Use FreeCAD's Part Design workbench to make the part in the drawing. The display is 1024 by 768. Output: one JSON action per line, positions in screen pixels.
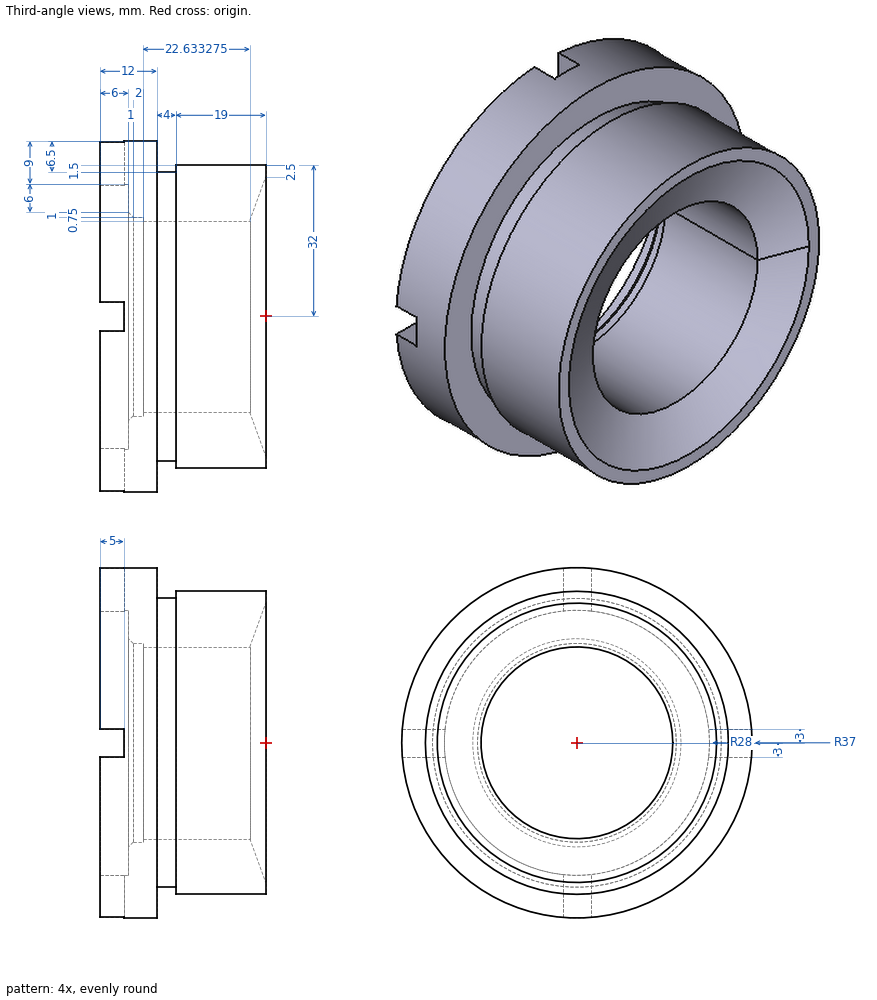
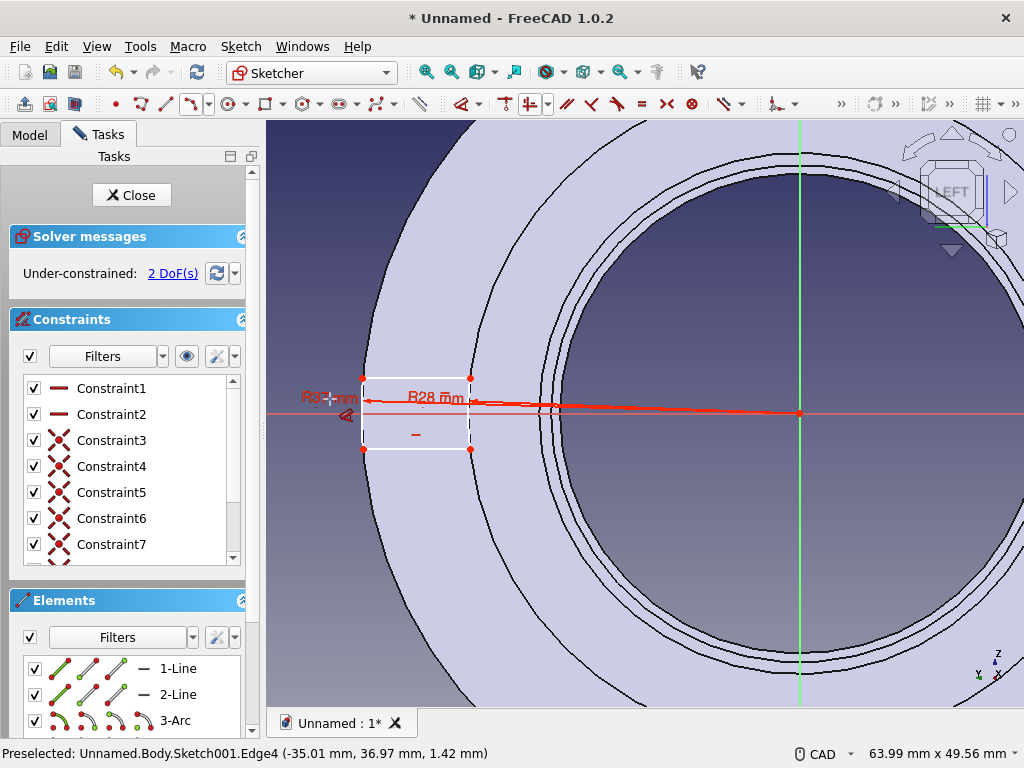
{"action": "left_click", "coordinate": [363, 449]}
{"action": "left_click", "coordinate": [834, 432]}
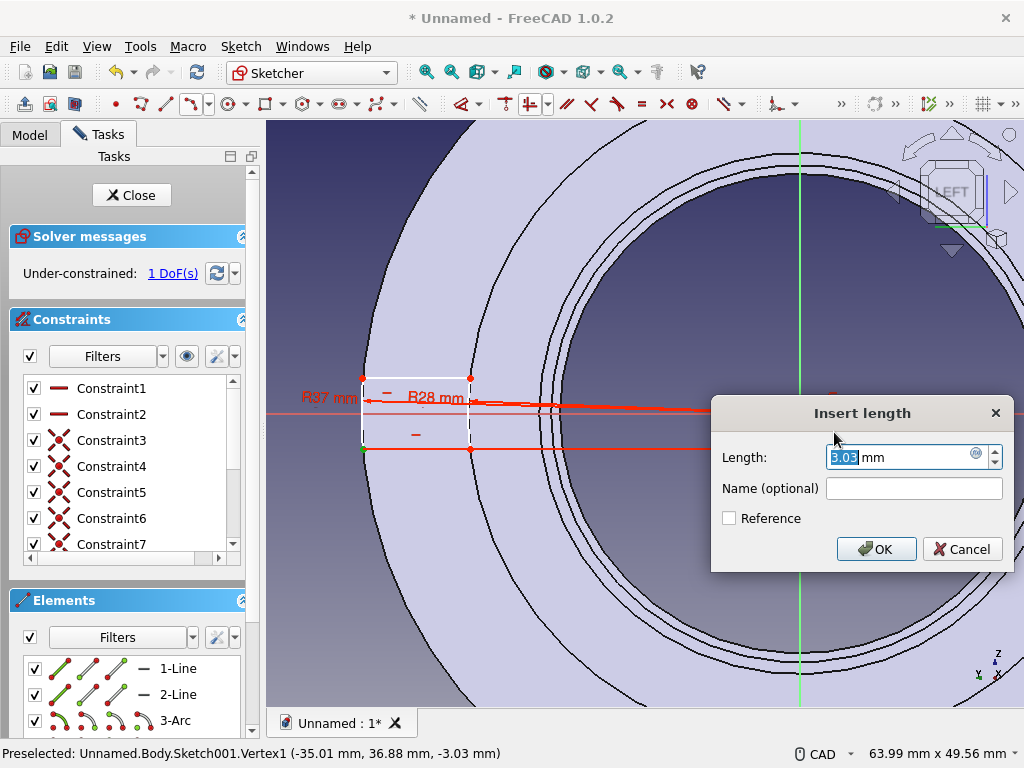
{"action": "type", "text": "3"}
{"action": "key", "text": "Return"}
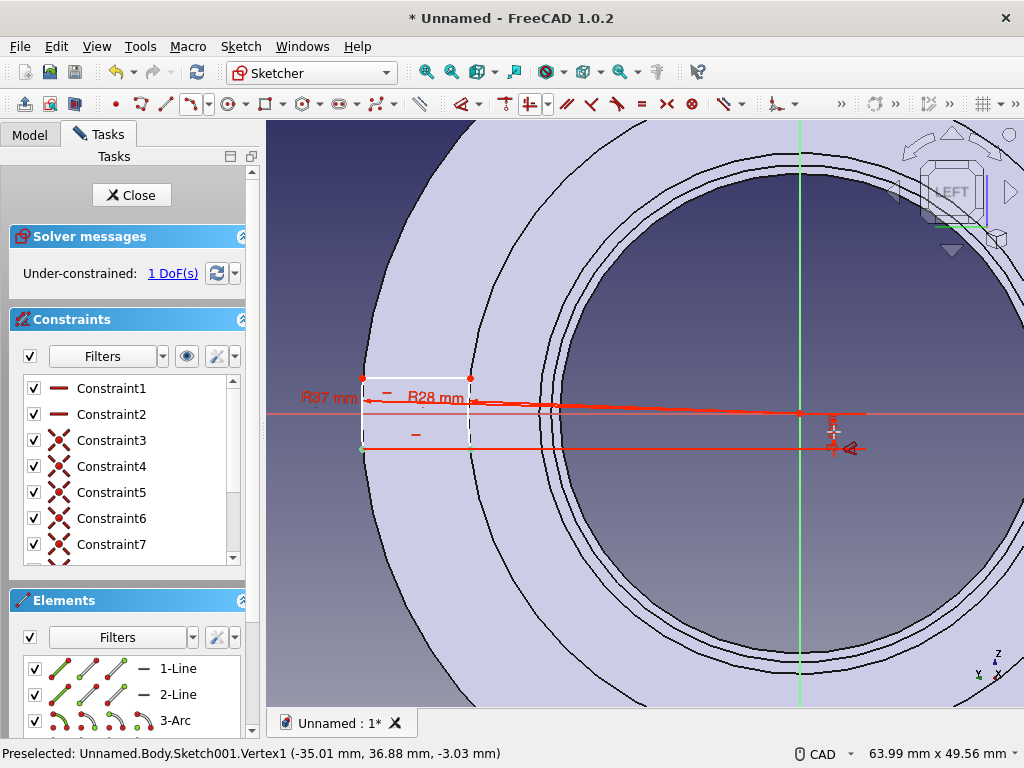
{"action": "left_click", "coordinate": [470, 378]}
{"action": "left_click", "coordinate": [834, 396]}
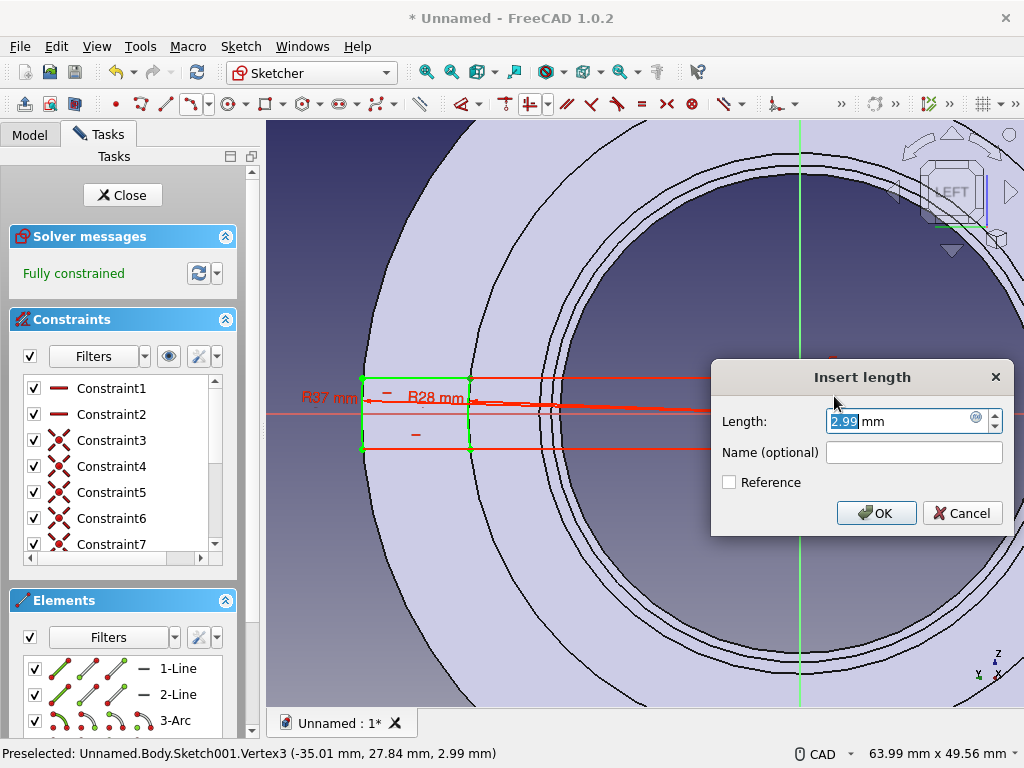
{"action": "type", "text": "3"}
{"action": "key", "text": "Return"}
{"action": "key", "text": "Escape"}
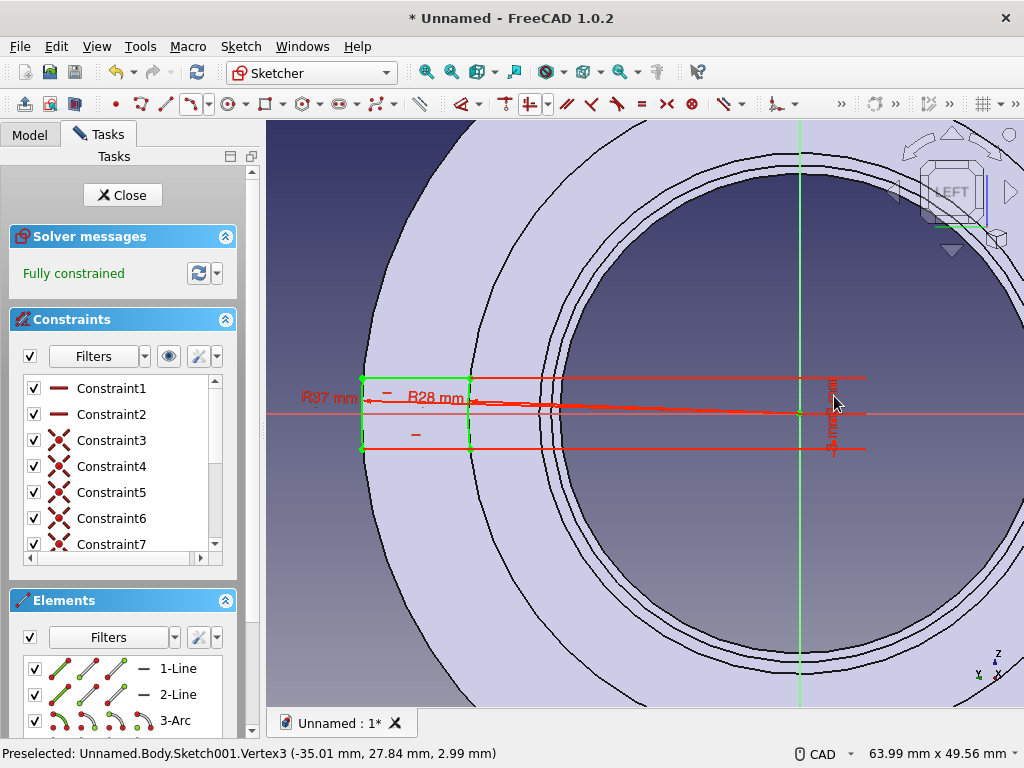
{"action": "left_click", "coordinate": [123, 195]}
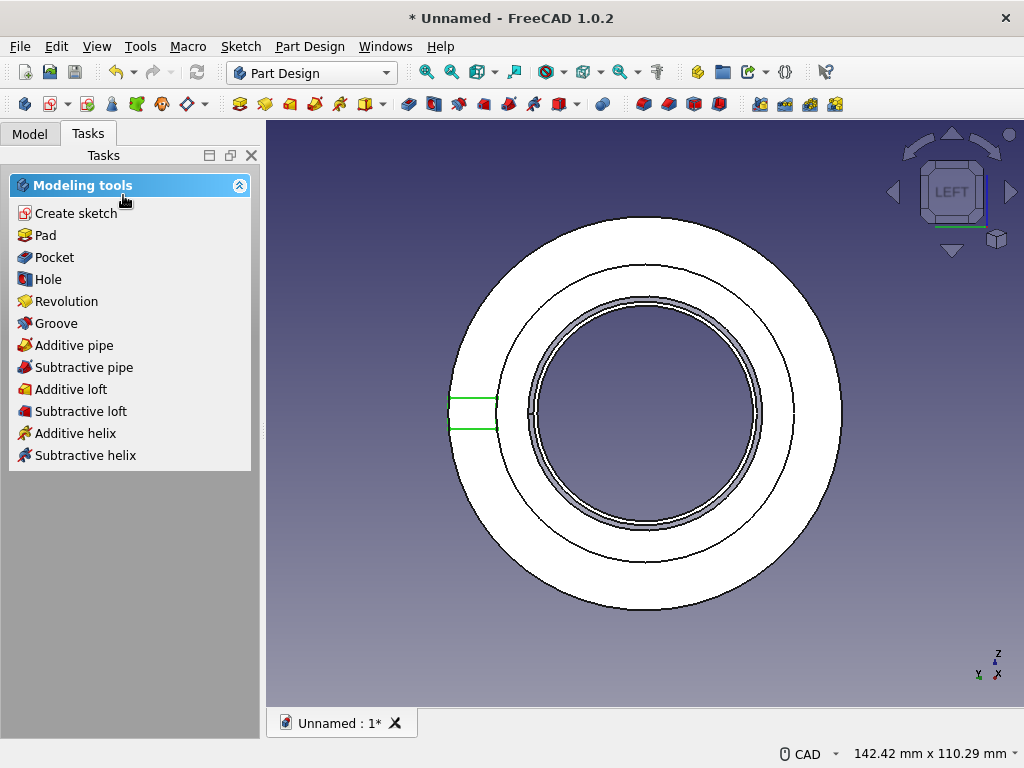
{"action": "left_click", "coordinate": [409, 104]}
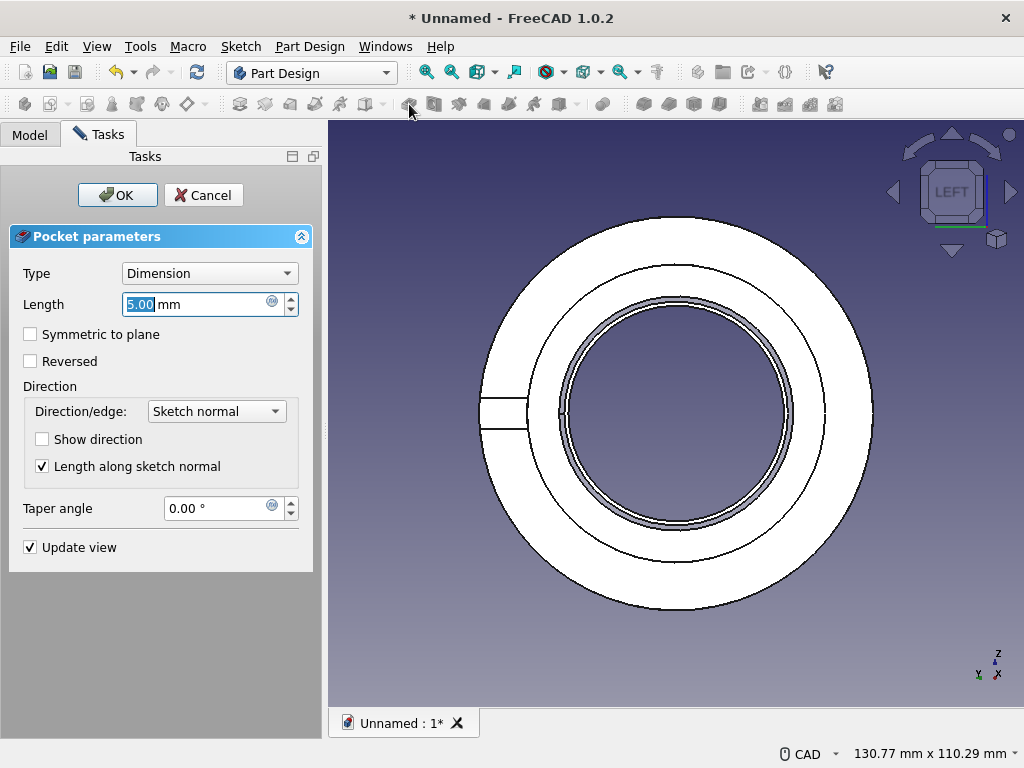
{"action": "type", "text": "5"}
{"action": "key", "text": "Tab"}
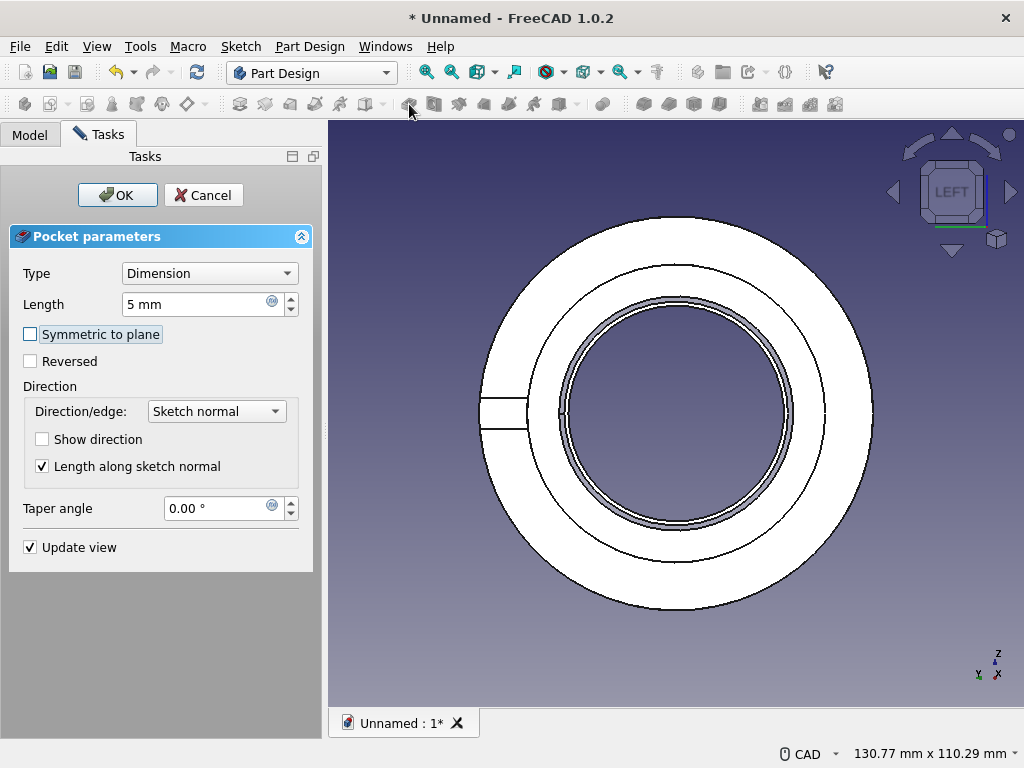
{"action": "left_click", "coordinate": [118, 195]}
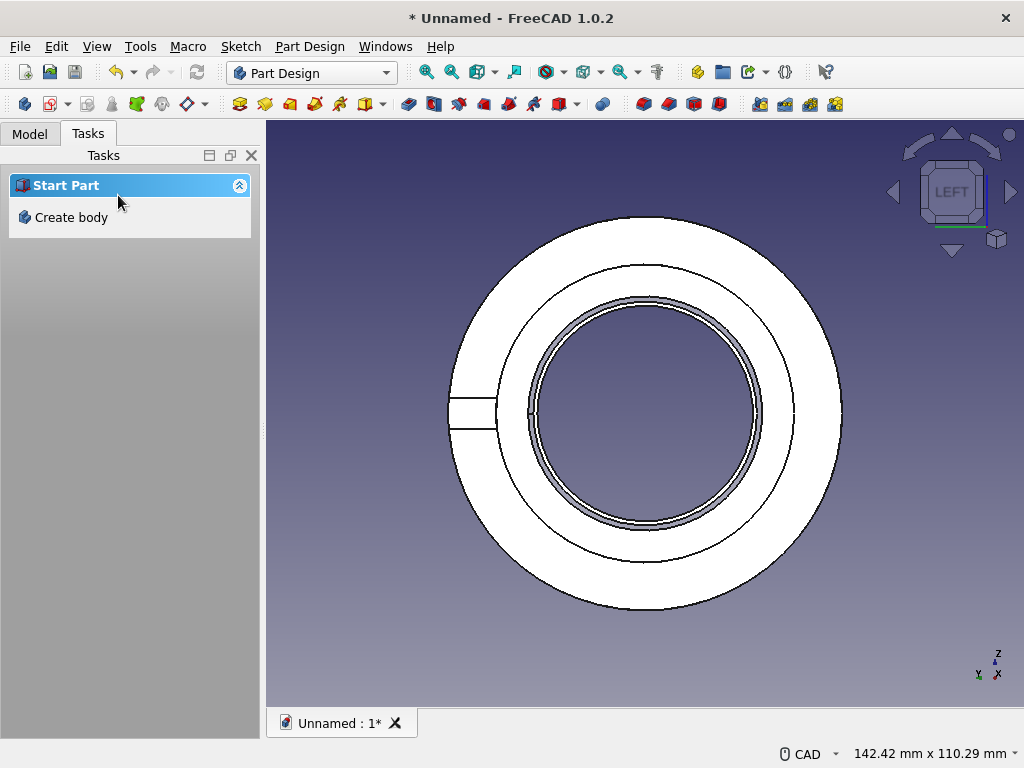
{"action": "left_click", "coordinate": [30, 134]}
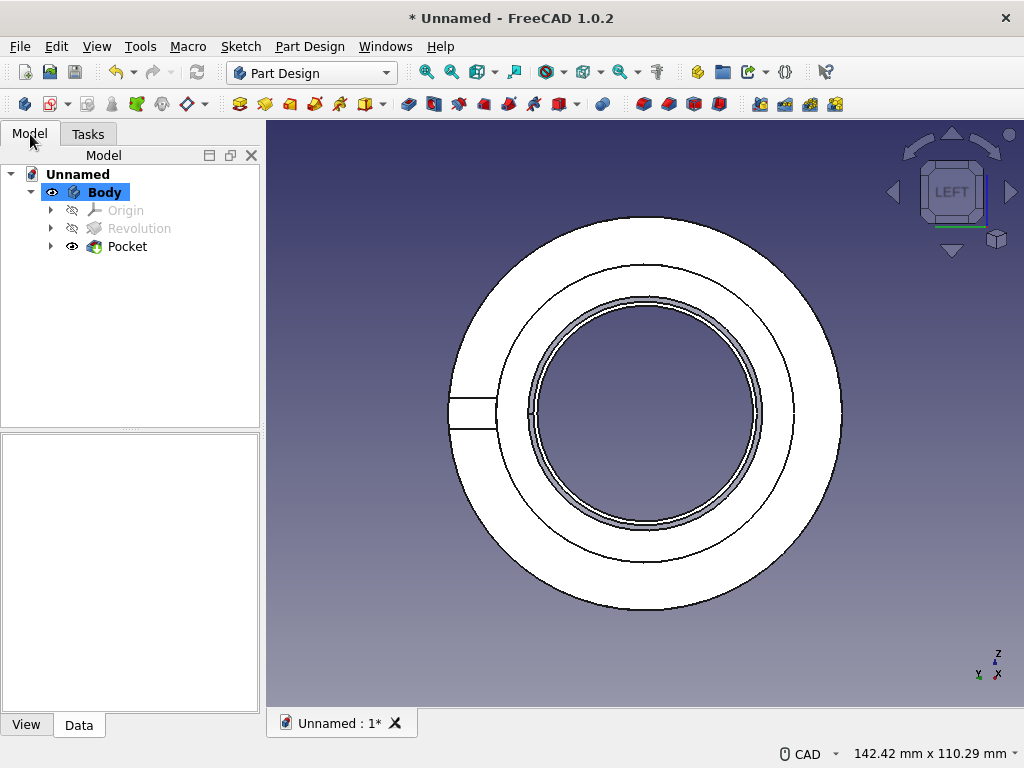
{"action": "left_click", "coordinate": [117, 246]}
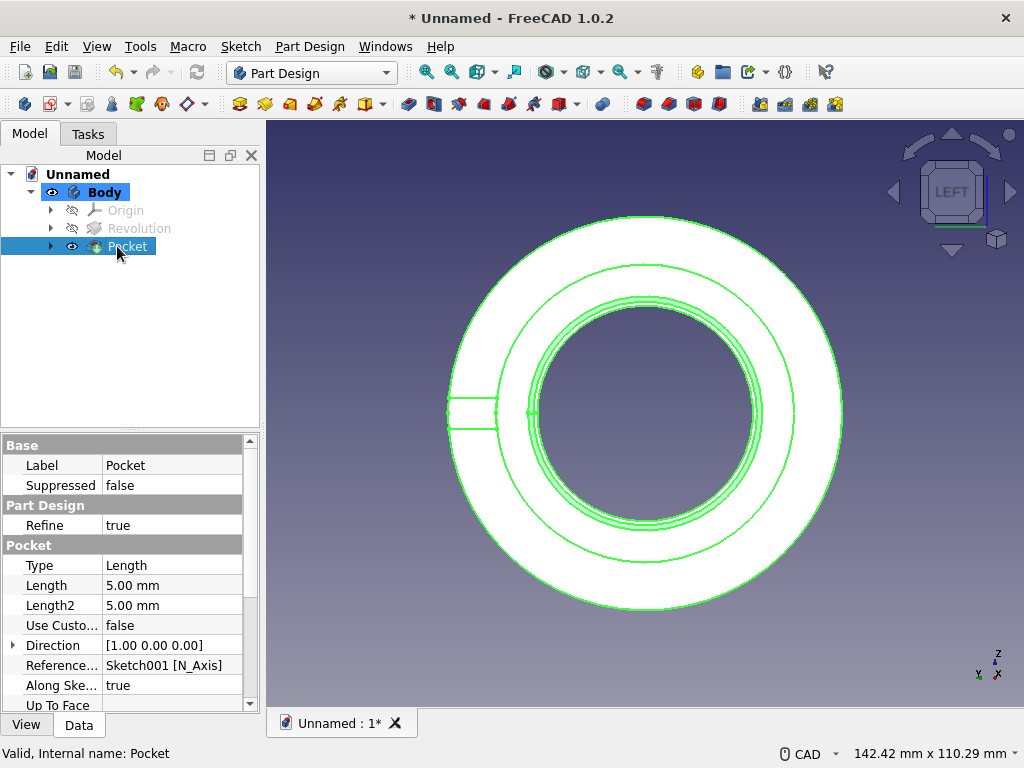
{"action": "left_click", "coordinate": [810, 104]}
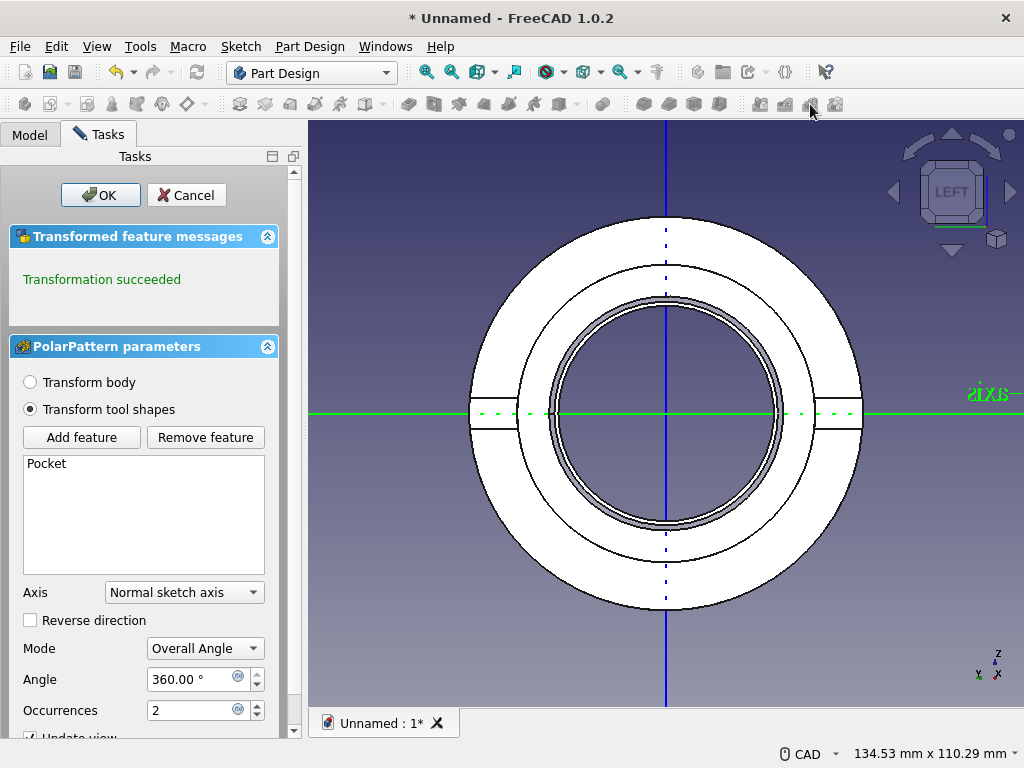
{"action": "left_click", "coordinate": [185, 592]}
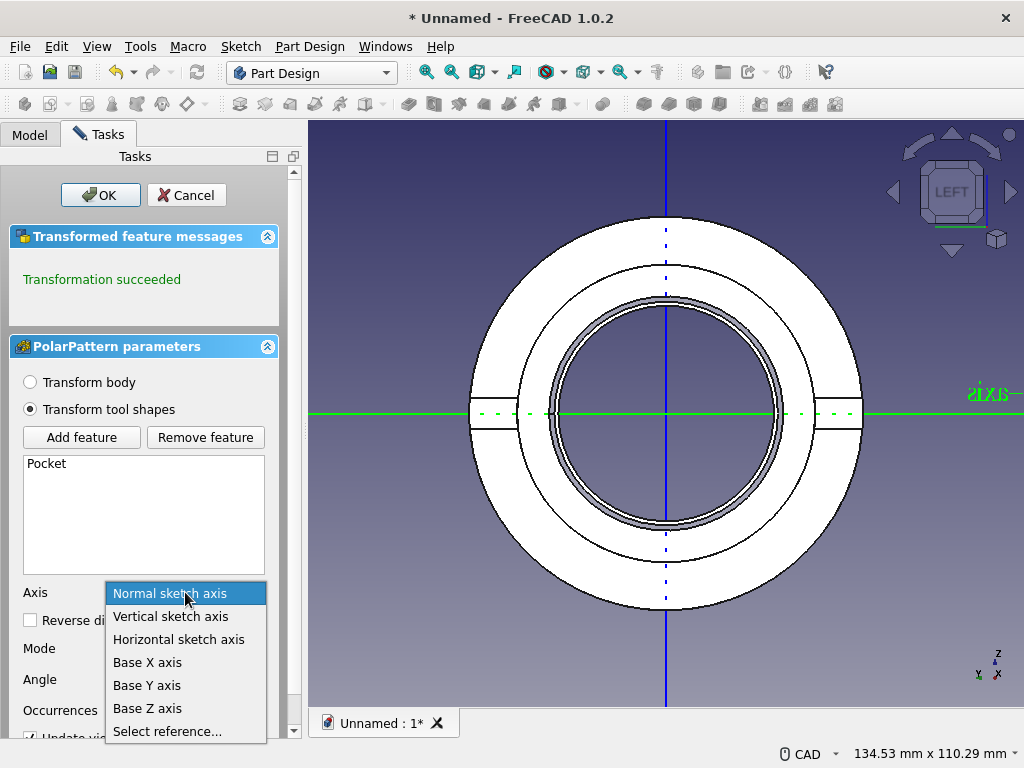
{"action": "left_click", "coordinate": [184, 662]}